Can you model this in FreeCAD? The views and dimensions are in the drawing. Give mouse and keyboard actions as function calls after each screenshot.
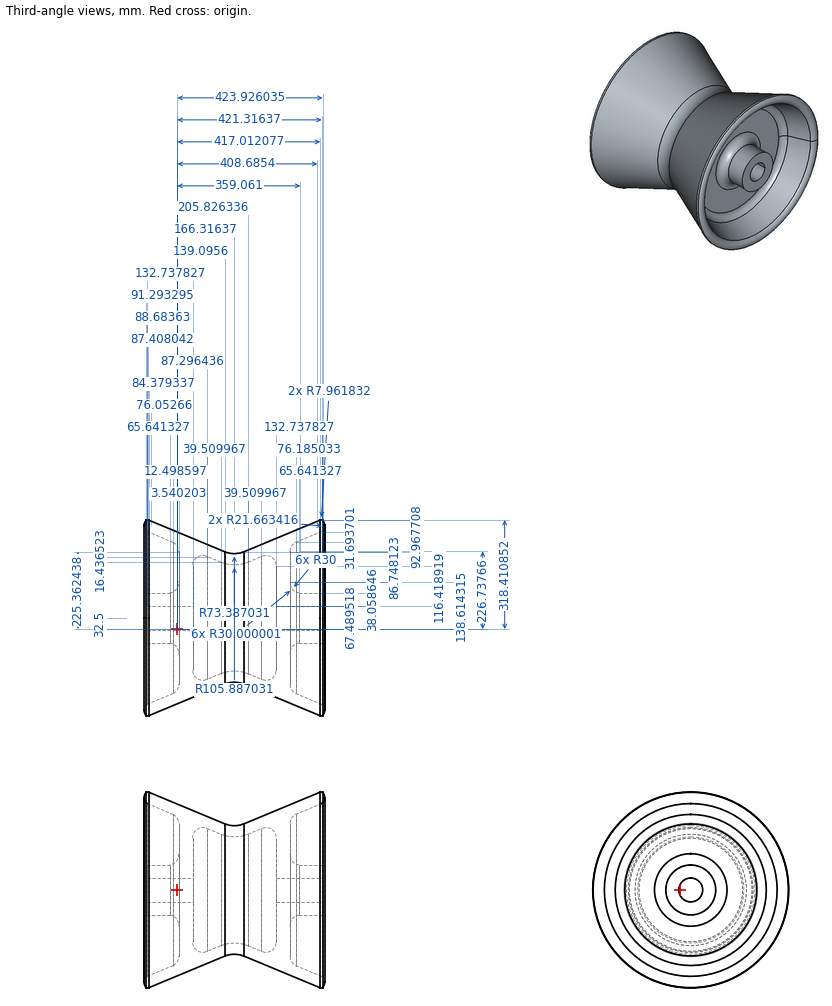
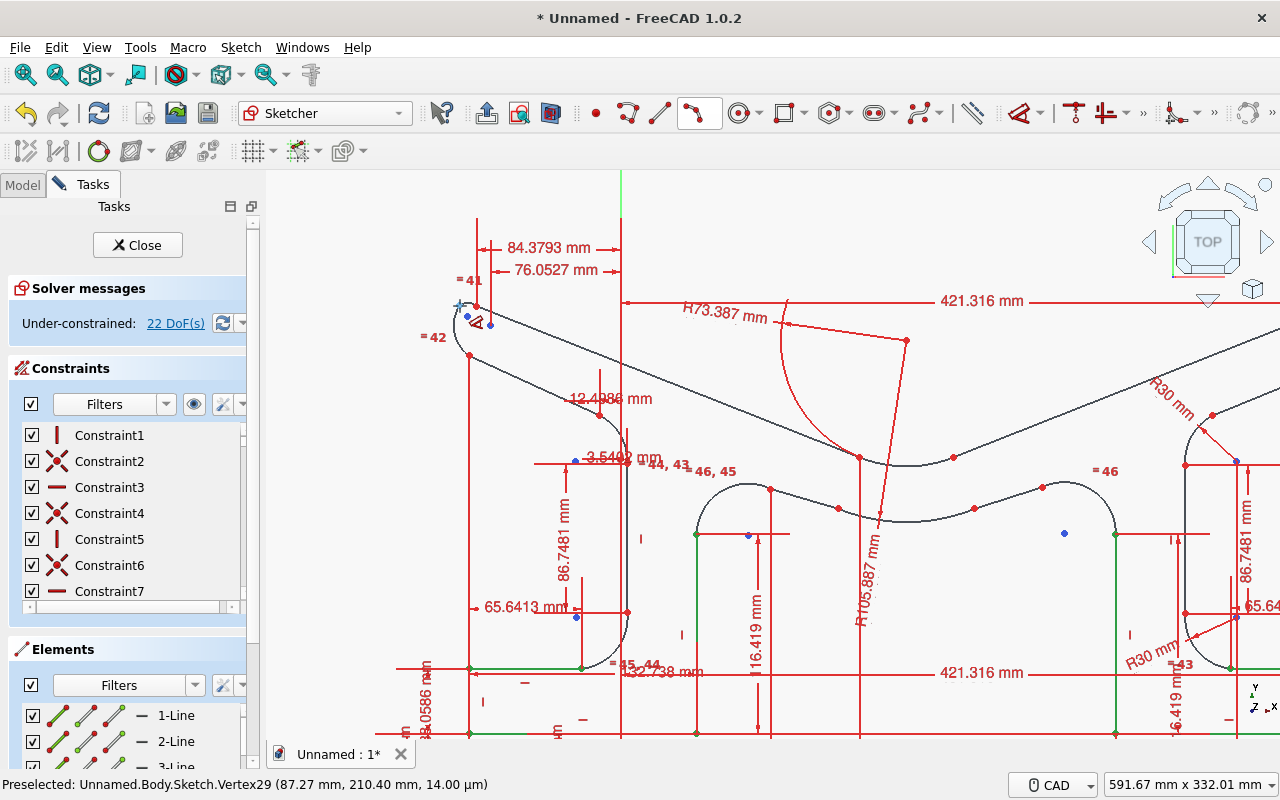
click(459, 306)
click(484, 272)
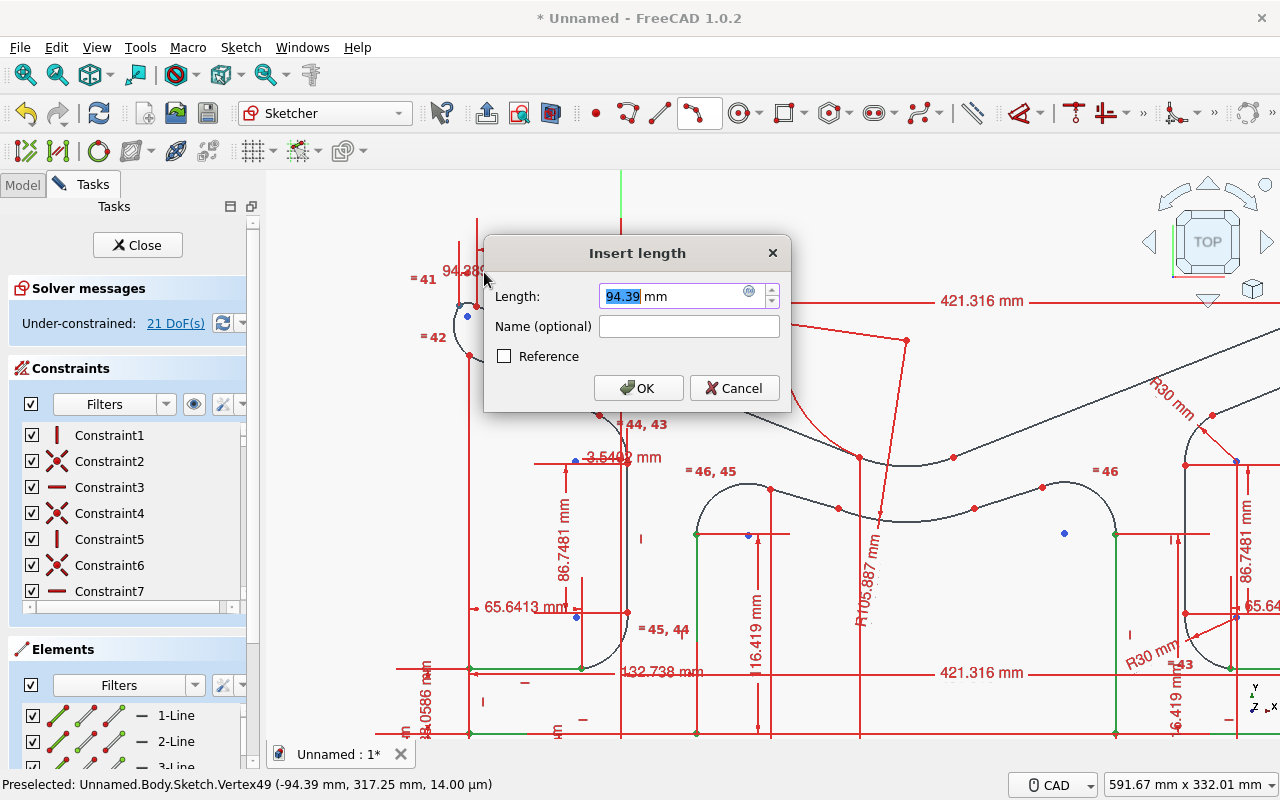
text(91.293295)
key(Return)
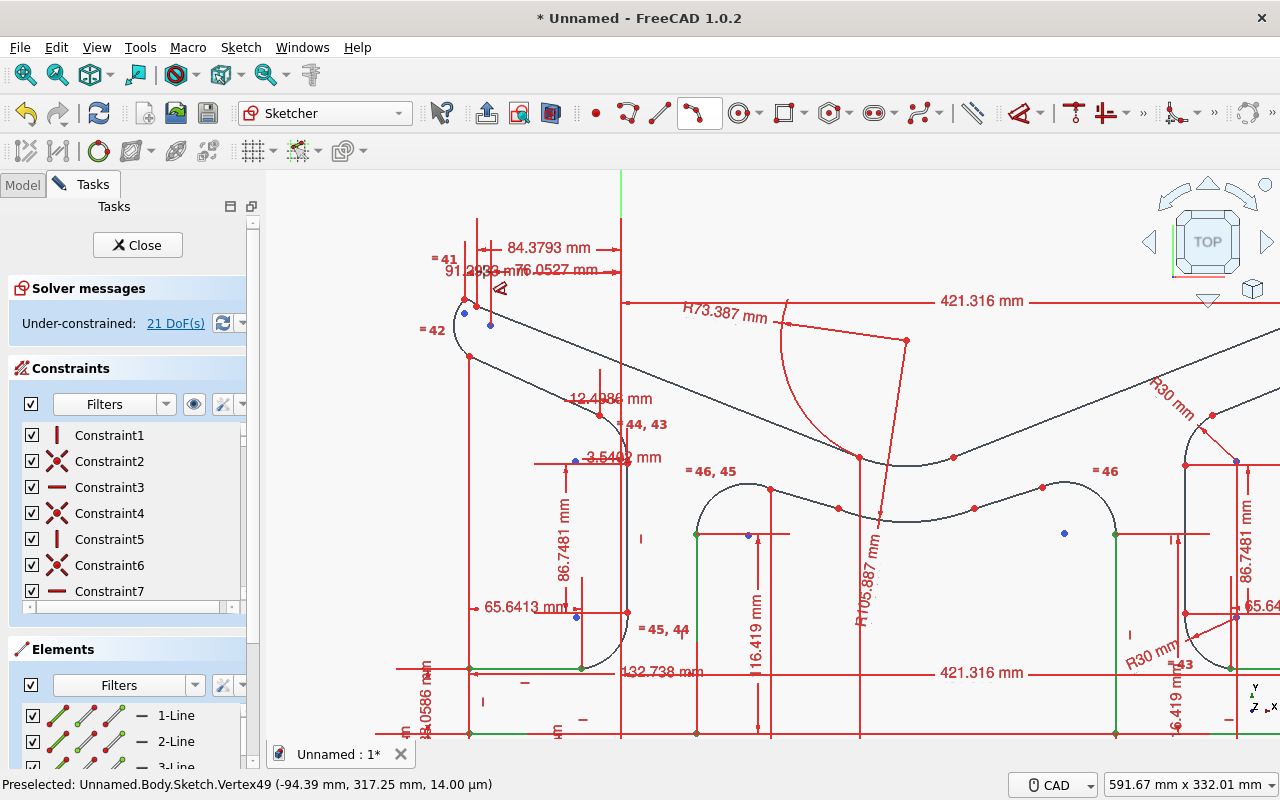
scroll(459, 306, down, 3)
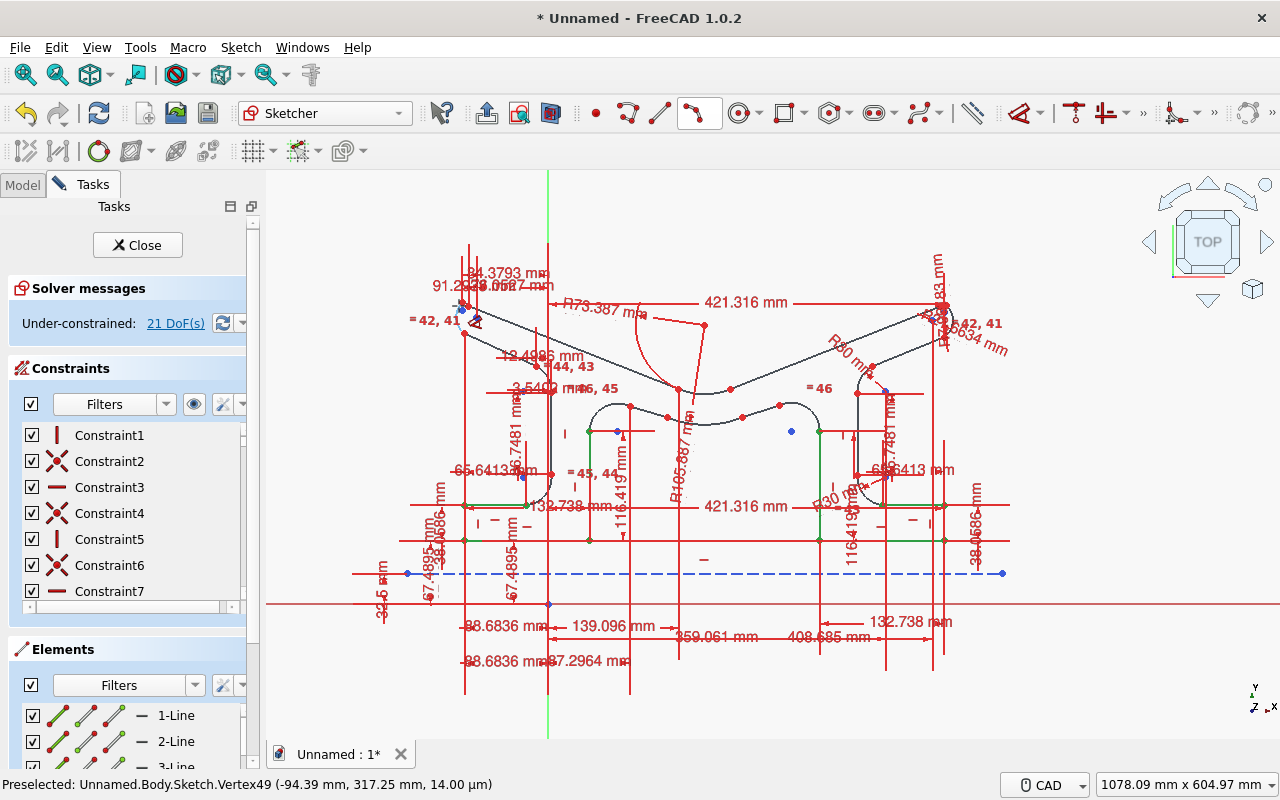
click(894, 358)
click(908, 400)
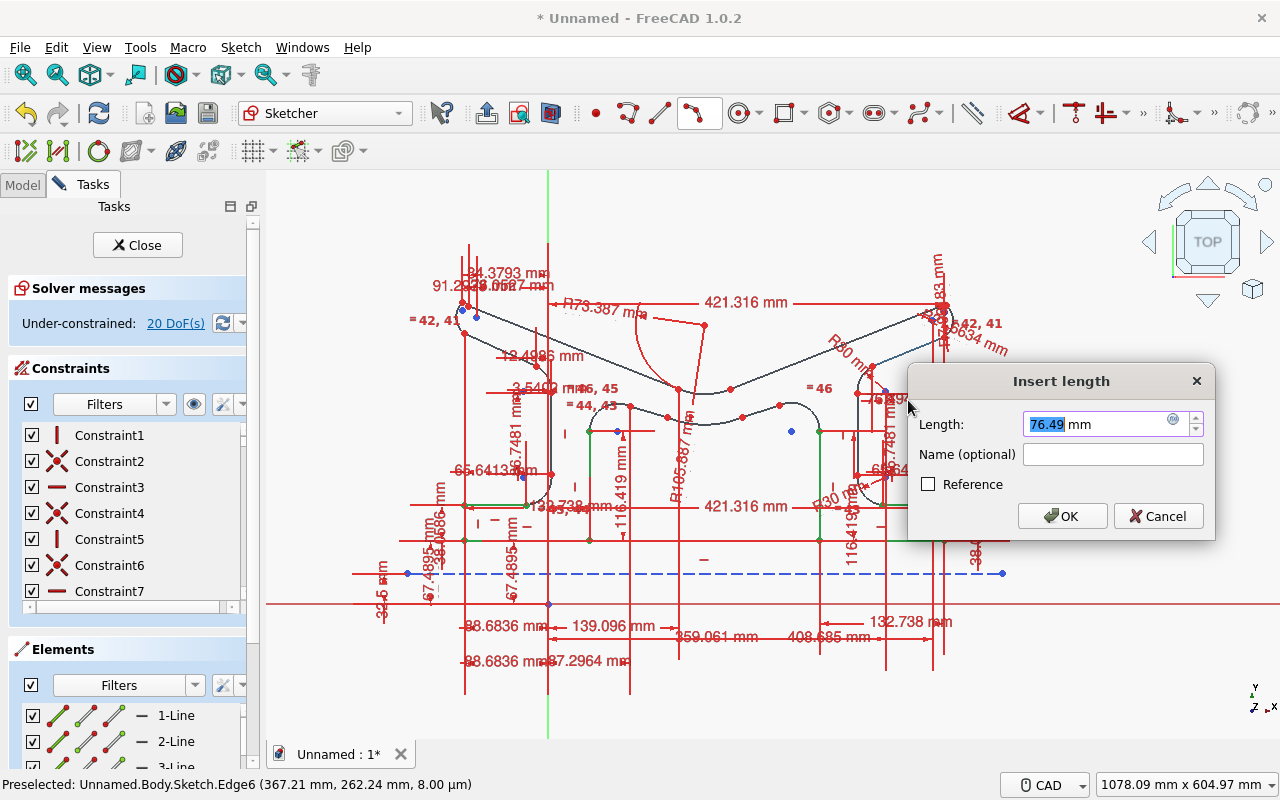
text(76.185033)
key(Return)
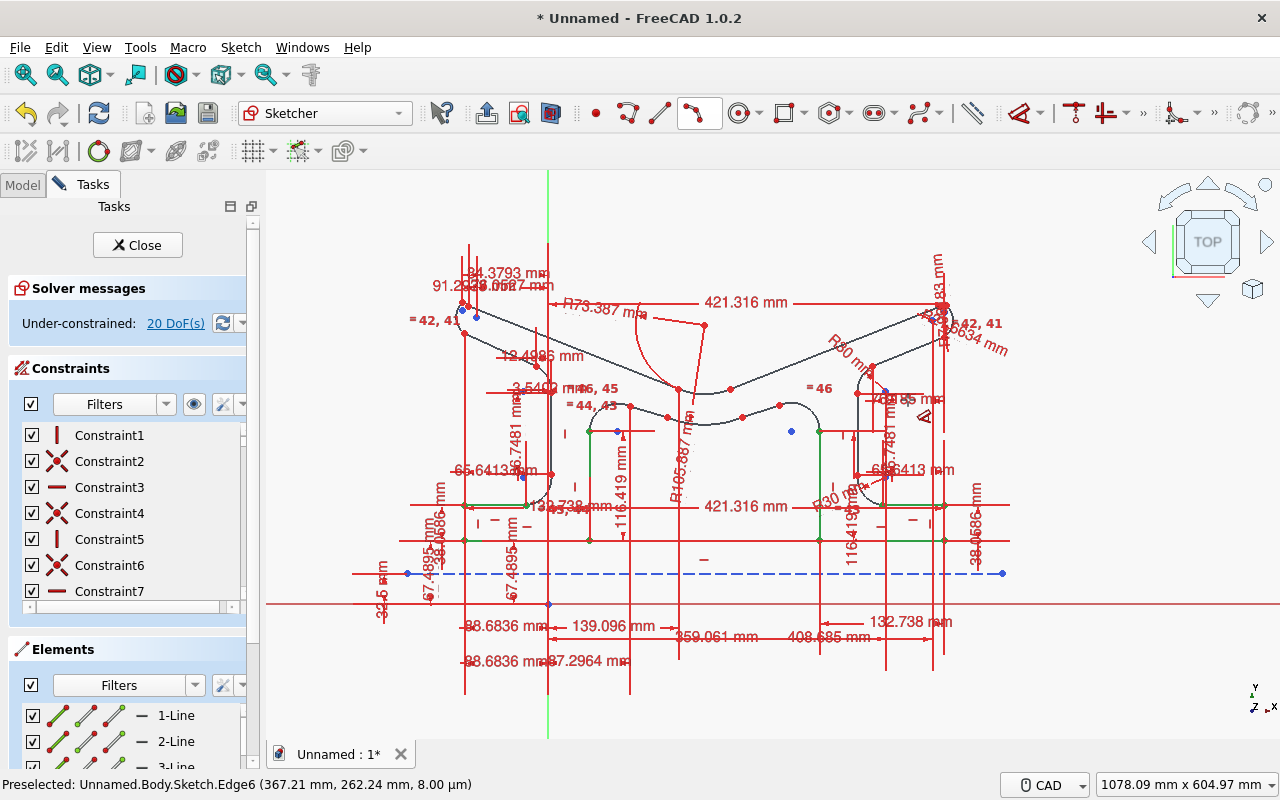
scroll(894, 357, up, 2)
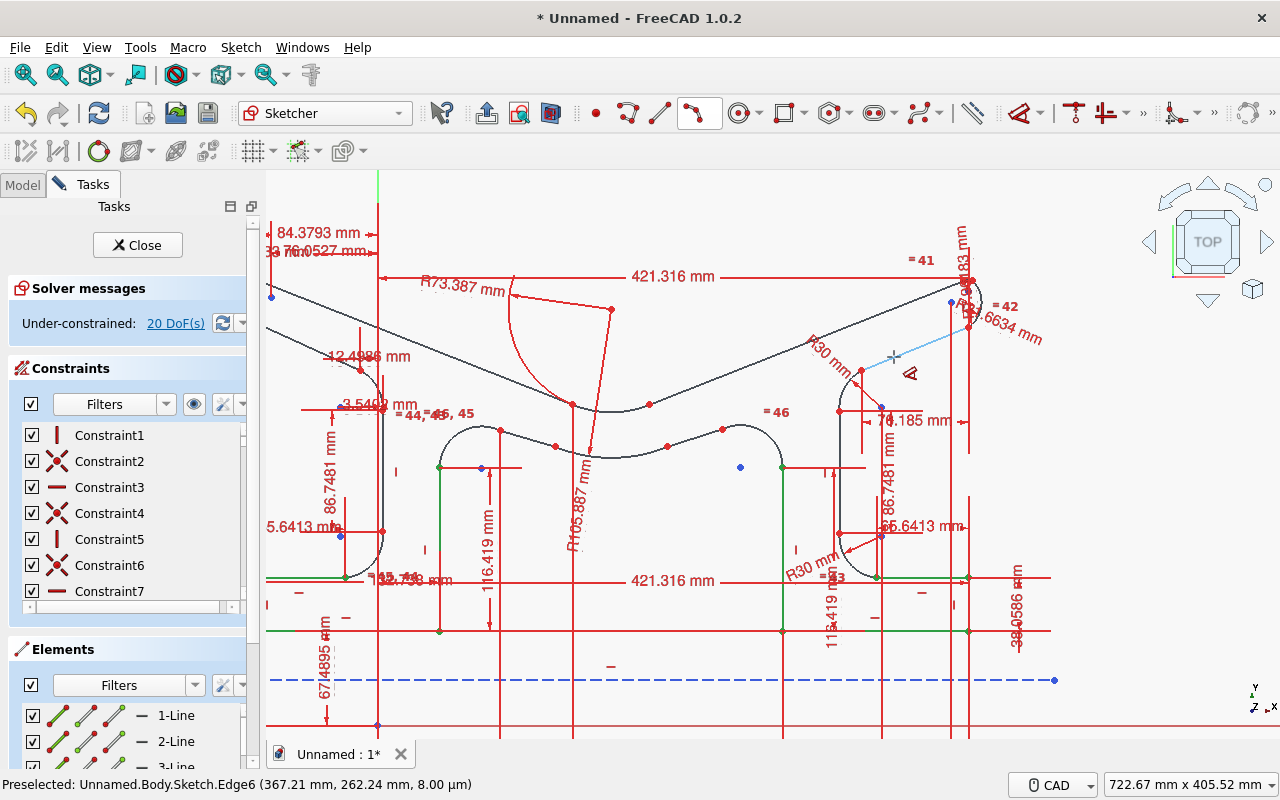
click(894, 358)
click(1003, 349)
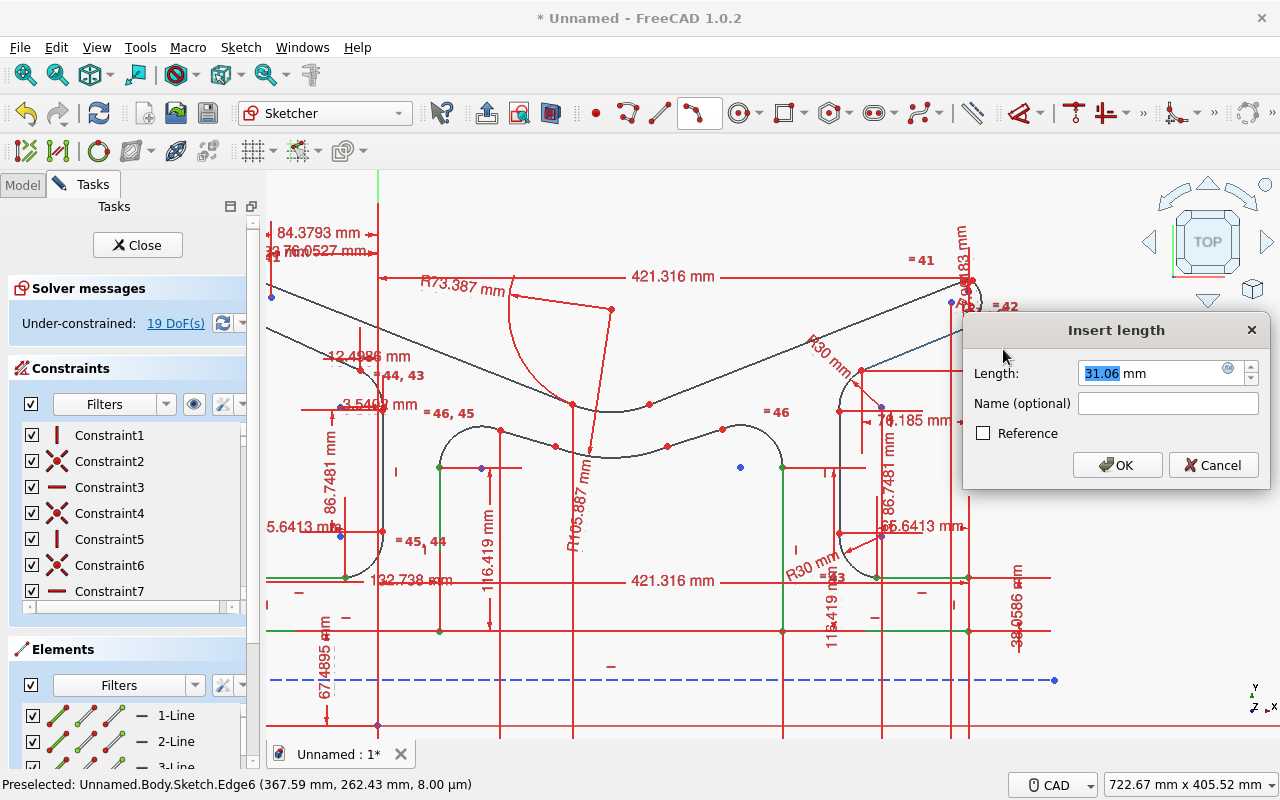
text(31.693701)
key(Return)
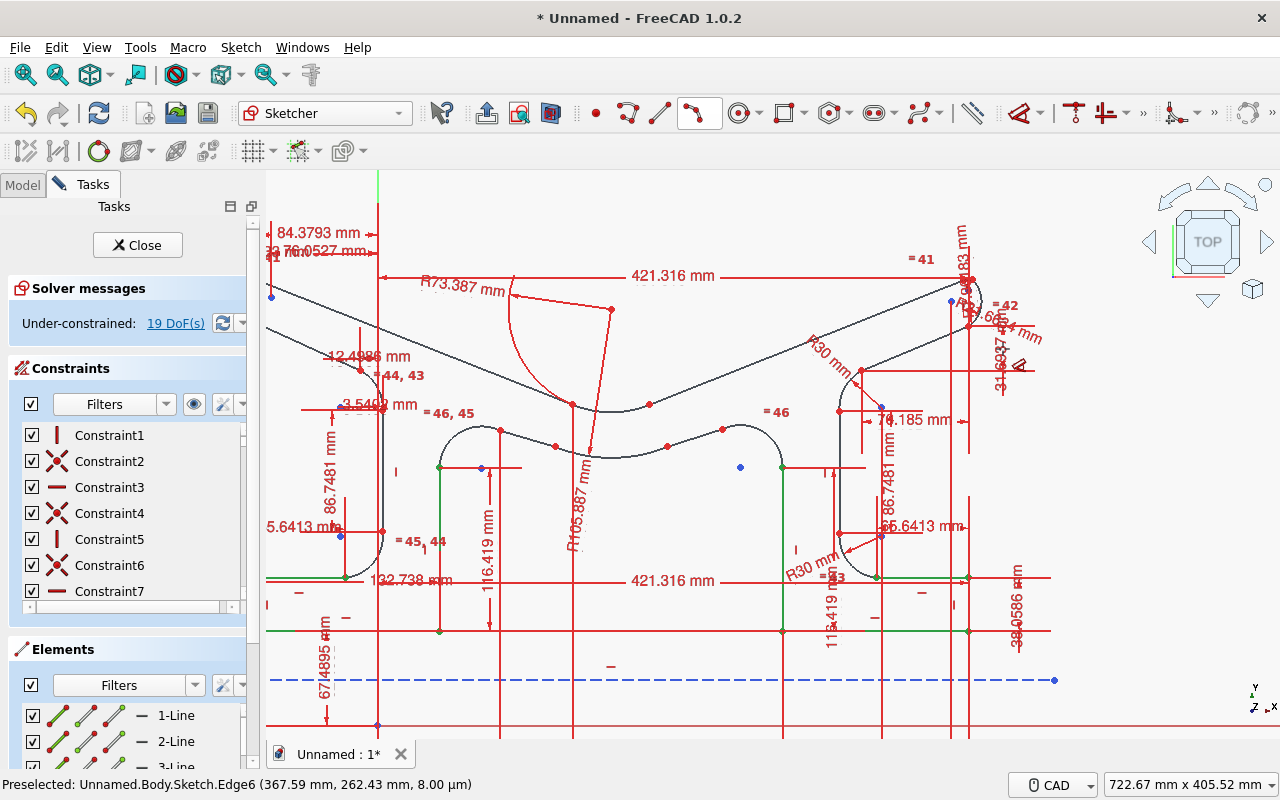
click(869, 318)
click(997, 371)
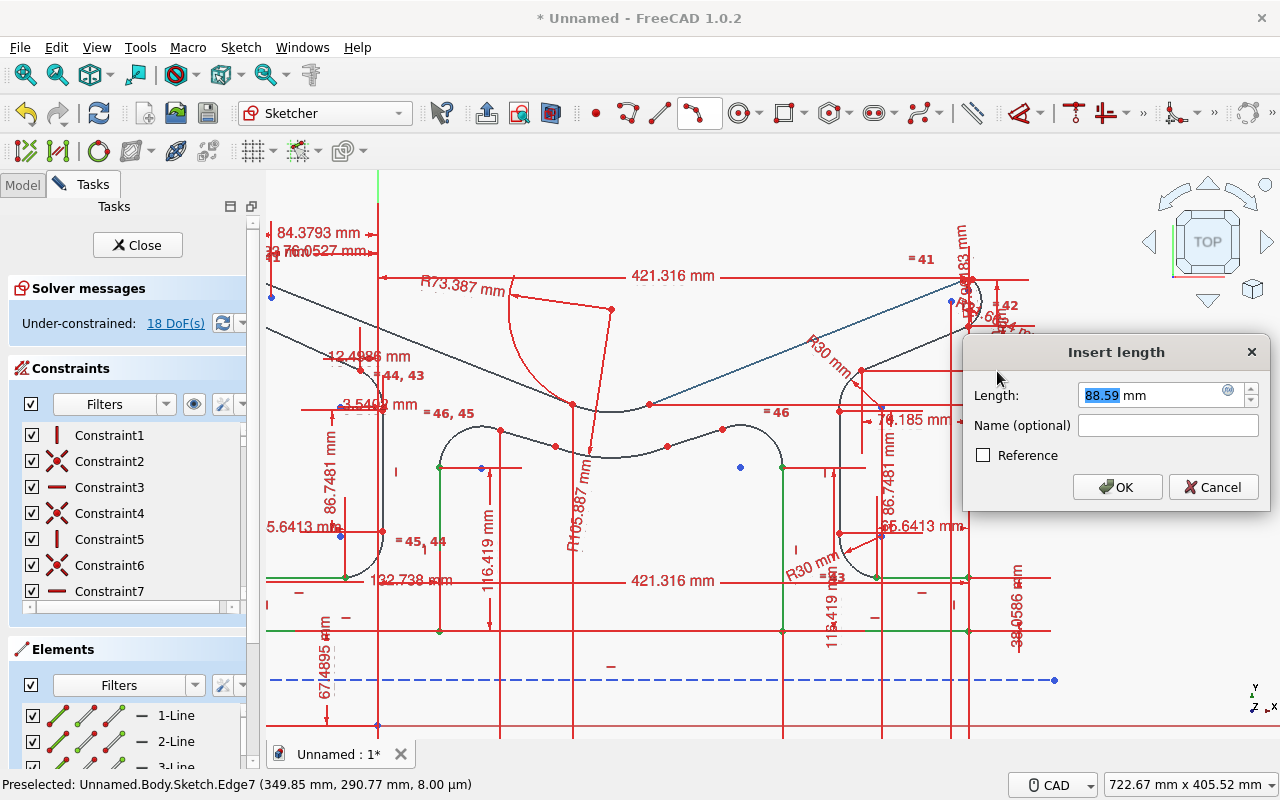
text(92.967708)
key(Return)